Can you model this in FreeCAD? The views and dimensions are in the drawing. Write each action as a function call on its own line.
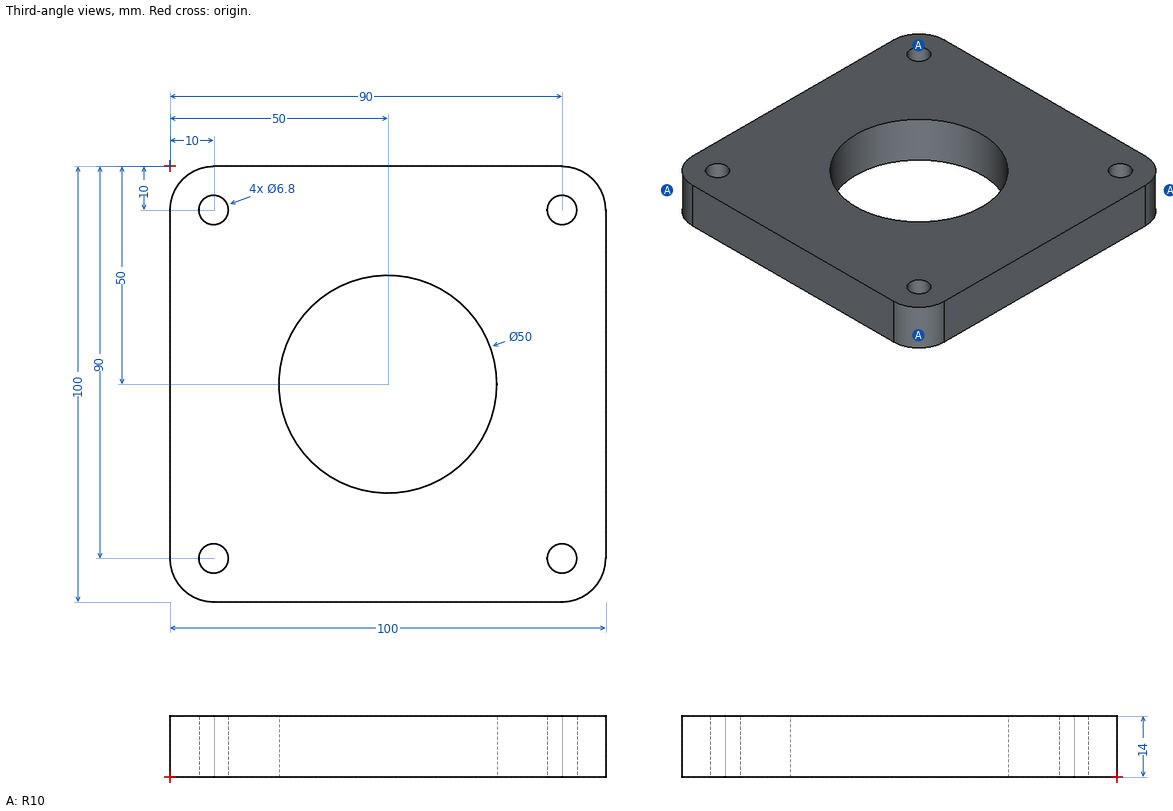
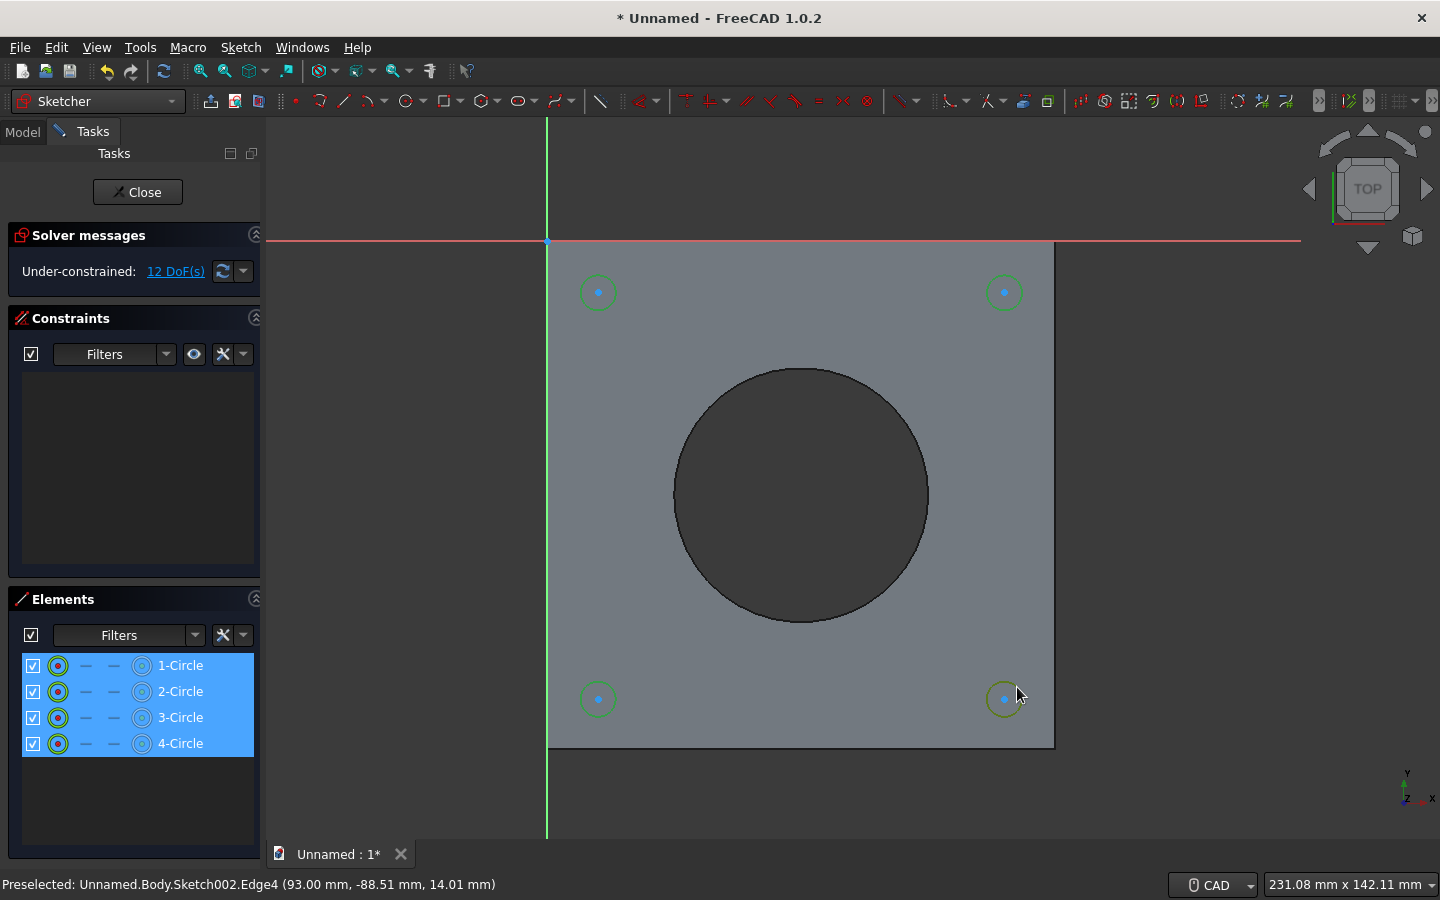
key(e)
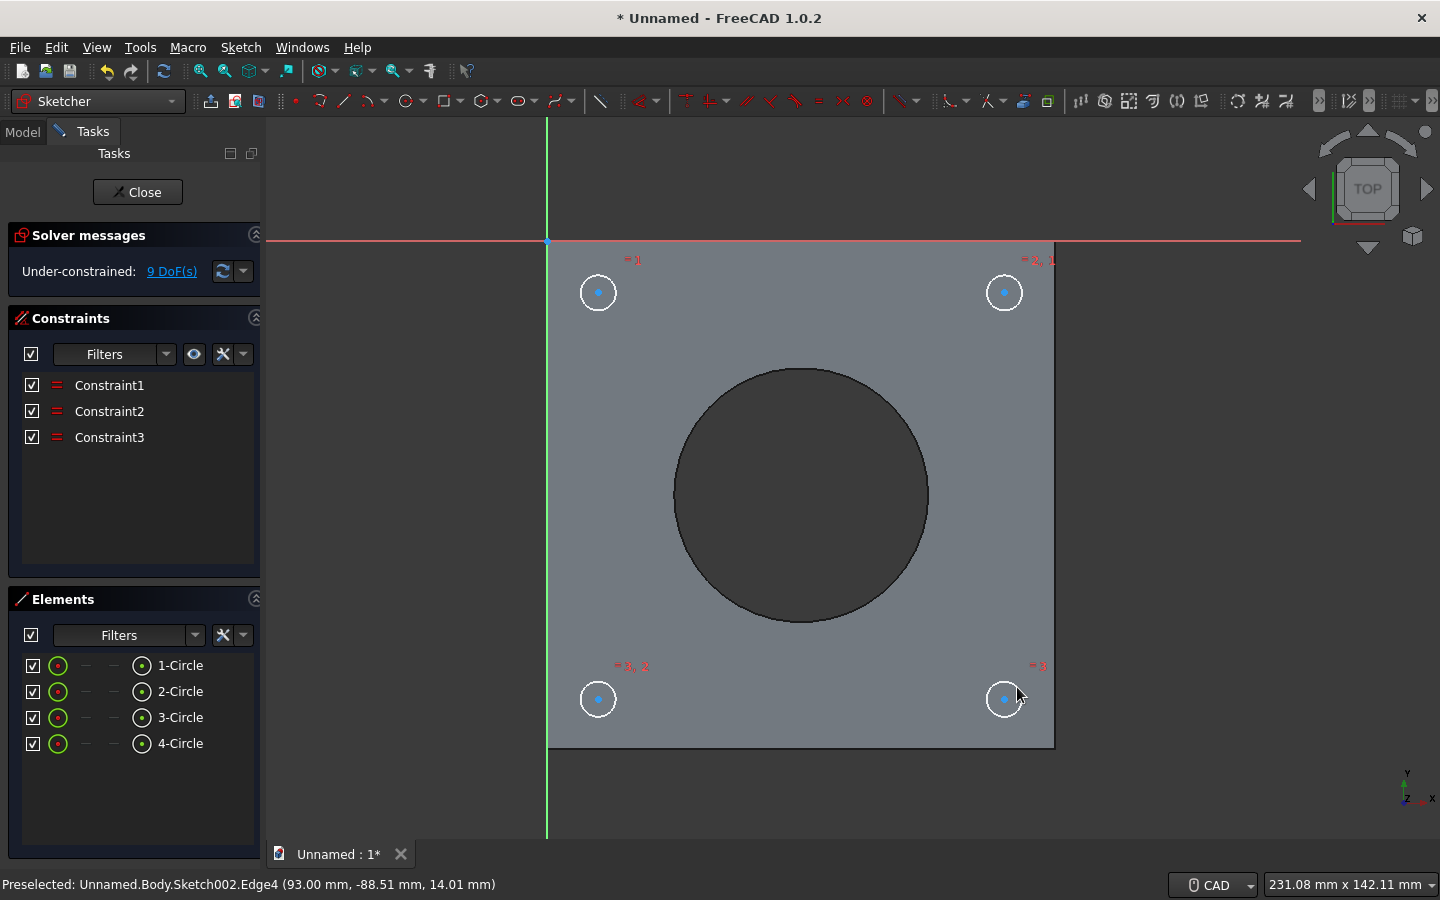
click(598, 293)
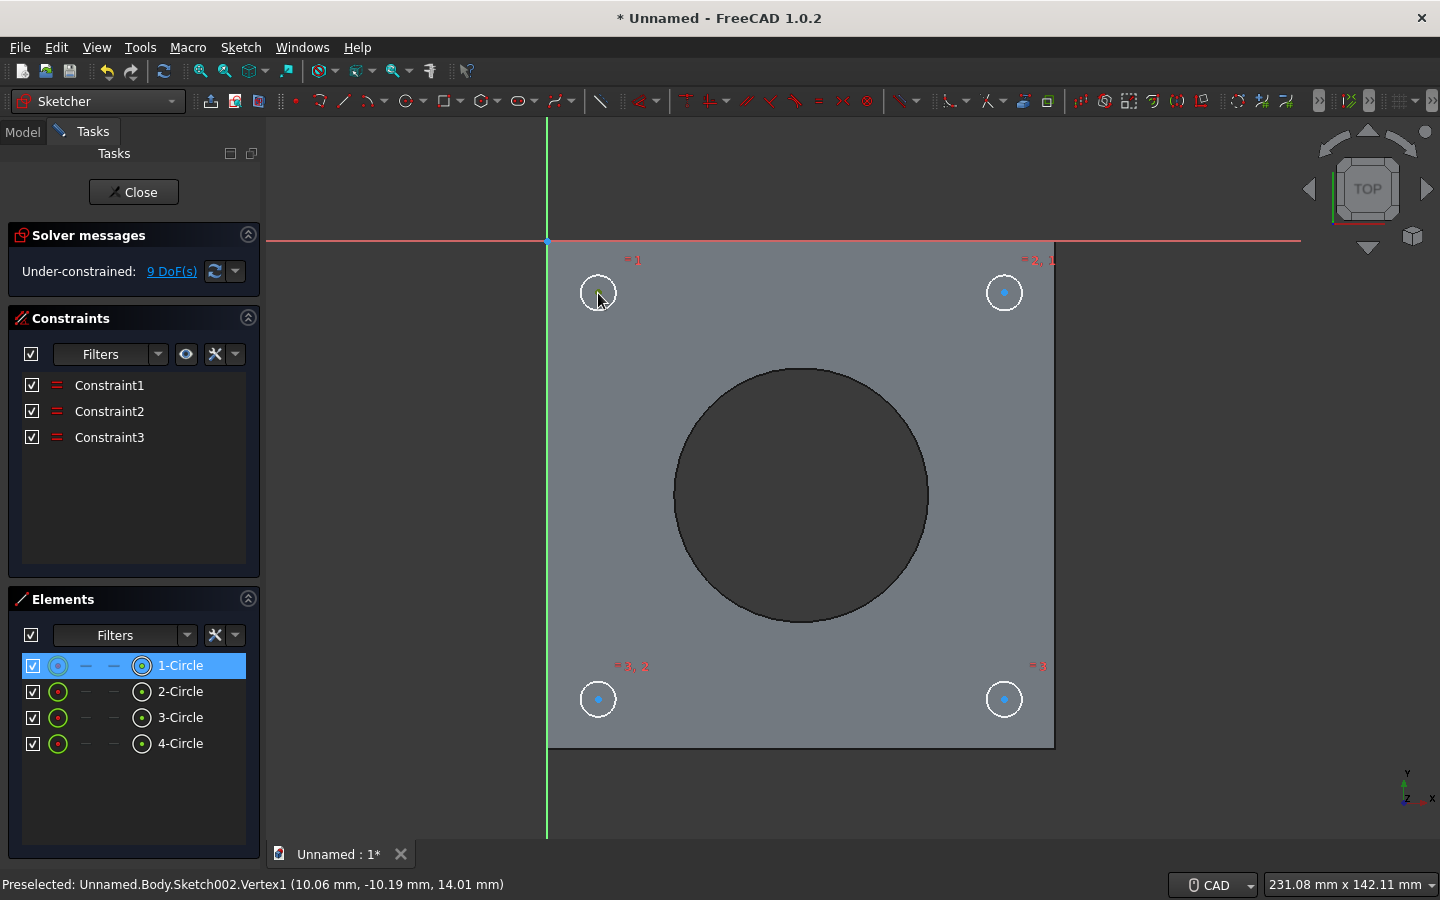
click(1005, 293)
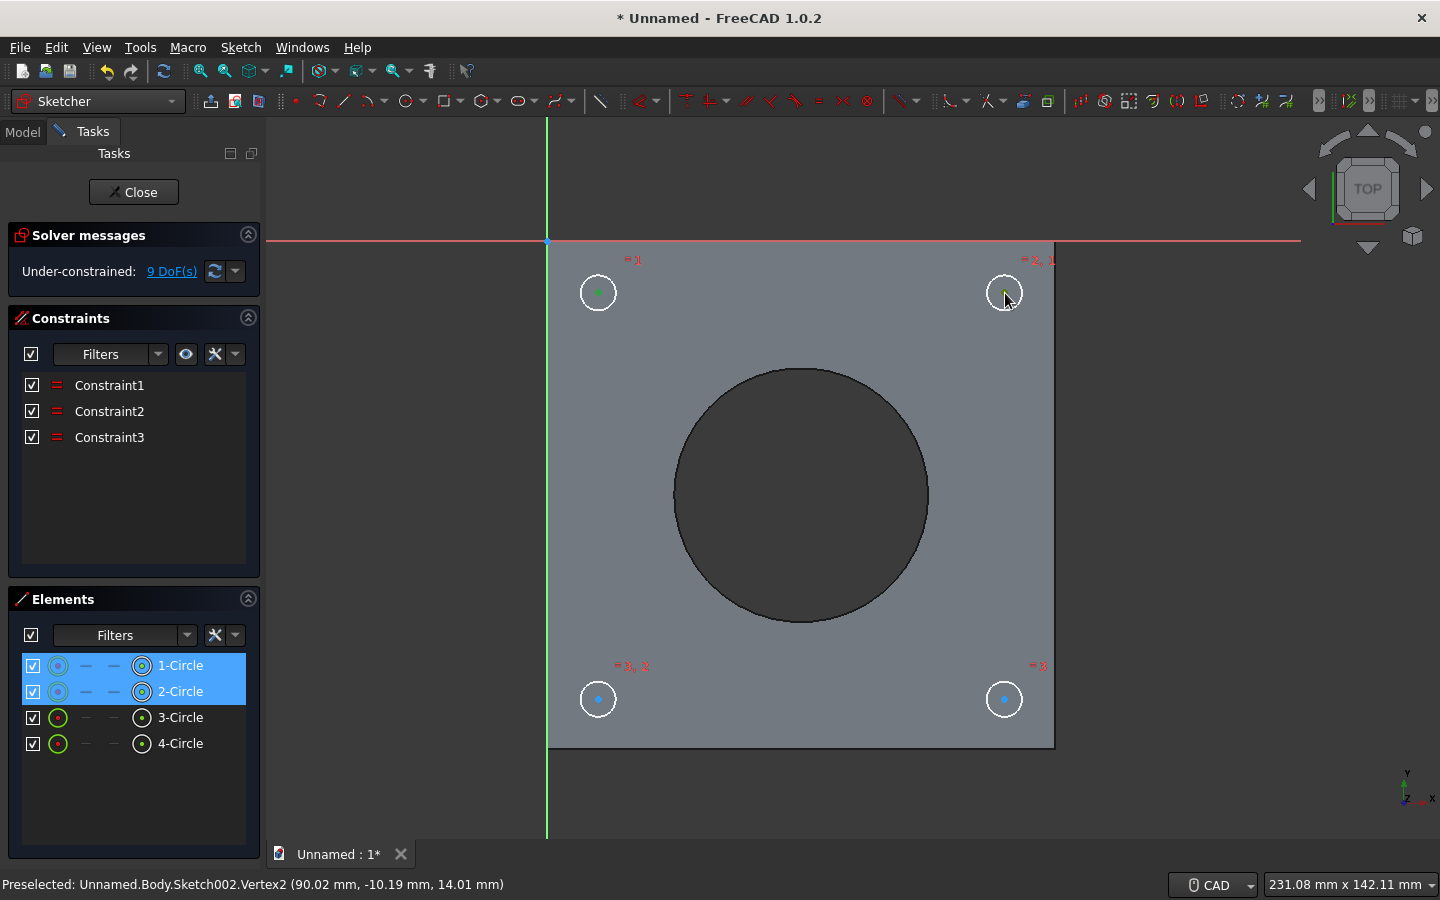
key(h)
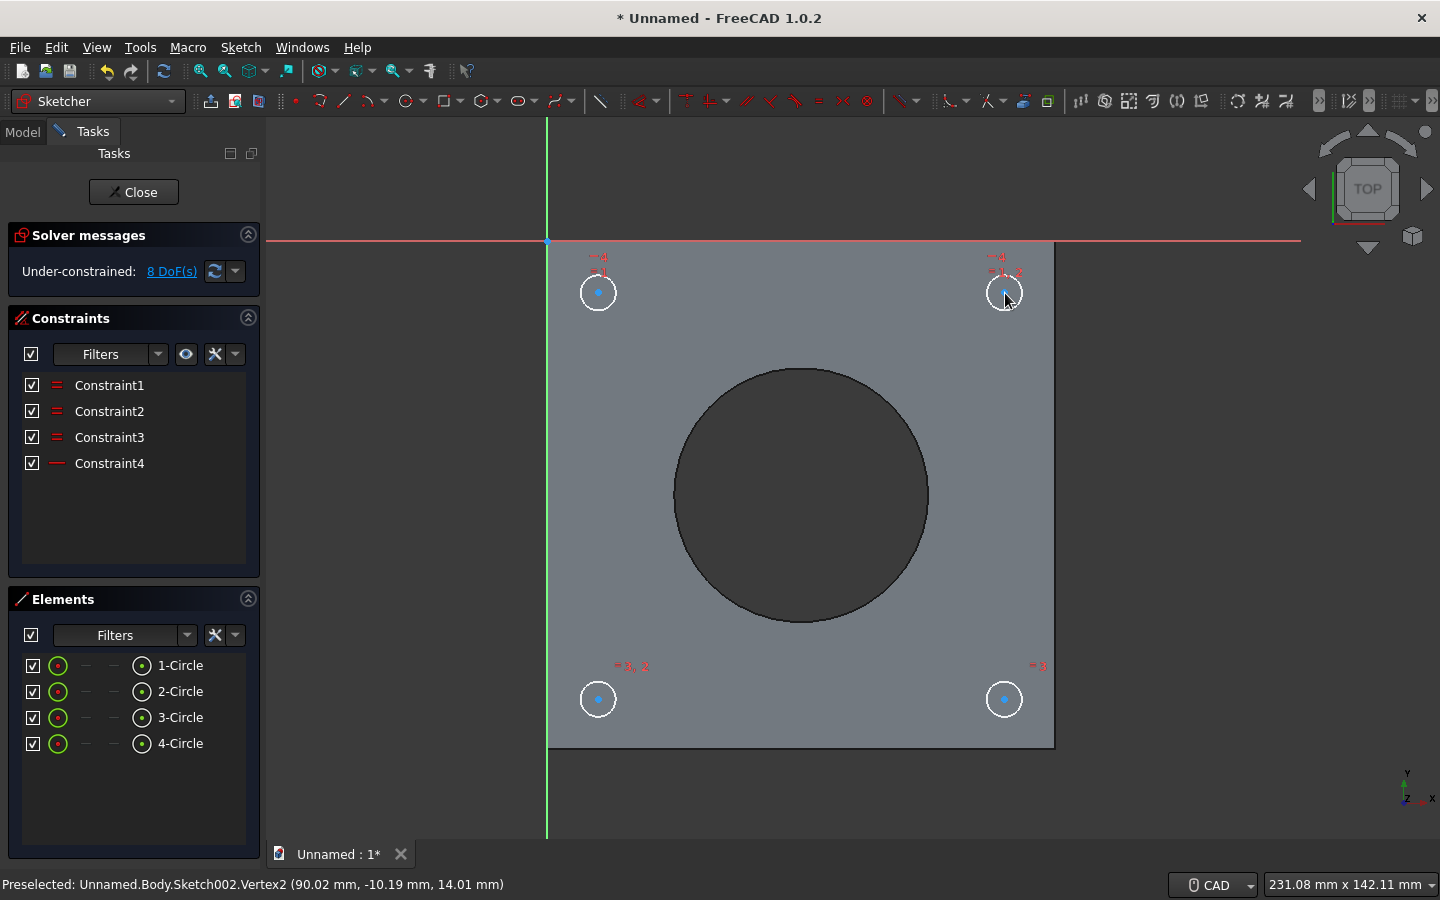
click(598, 293)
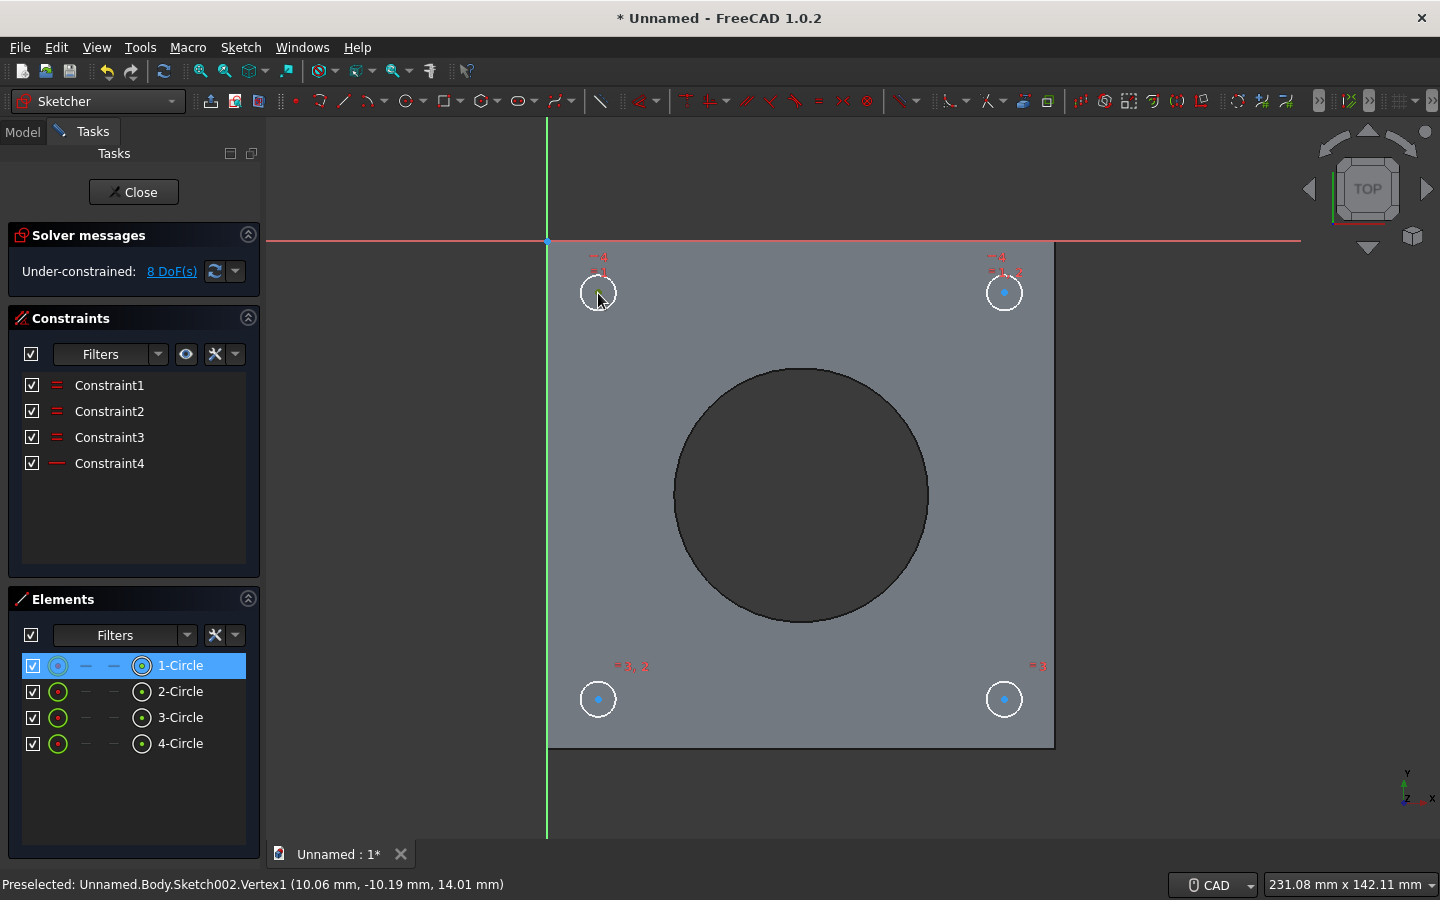
click(598, 699)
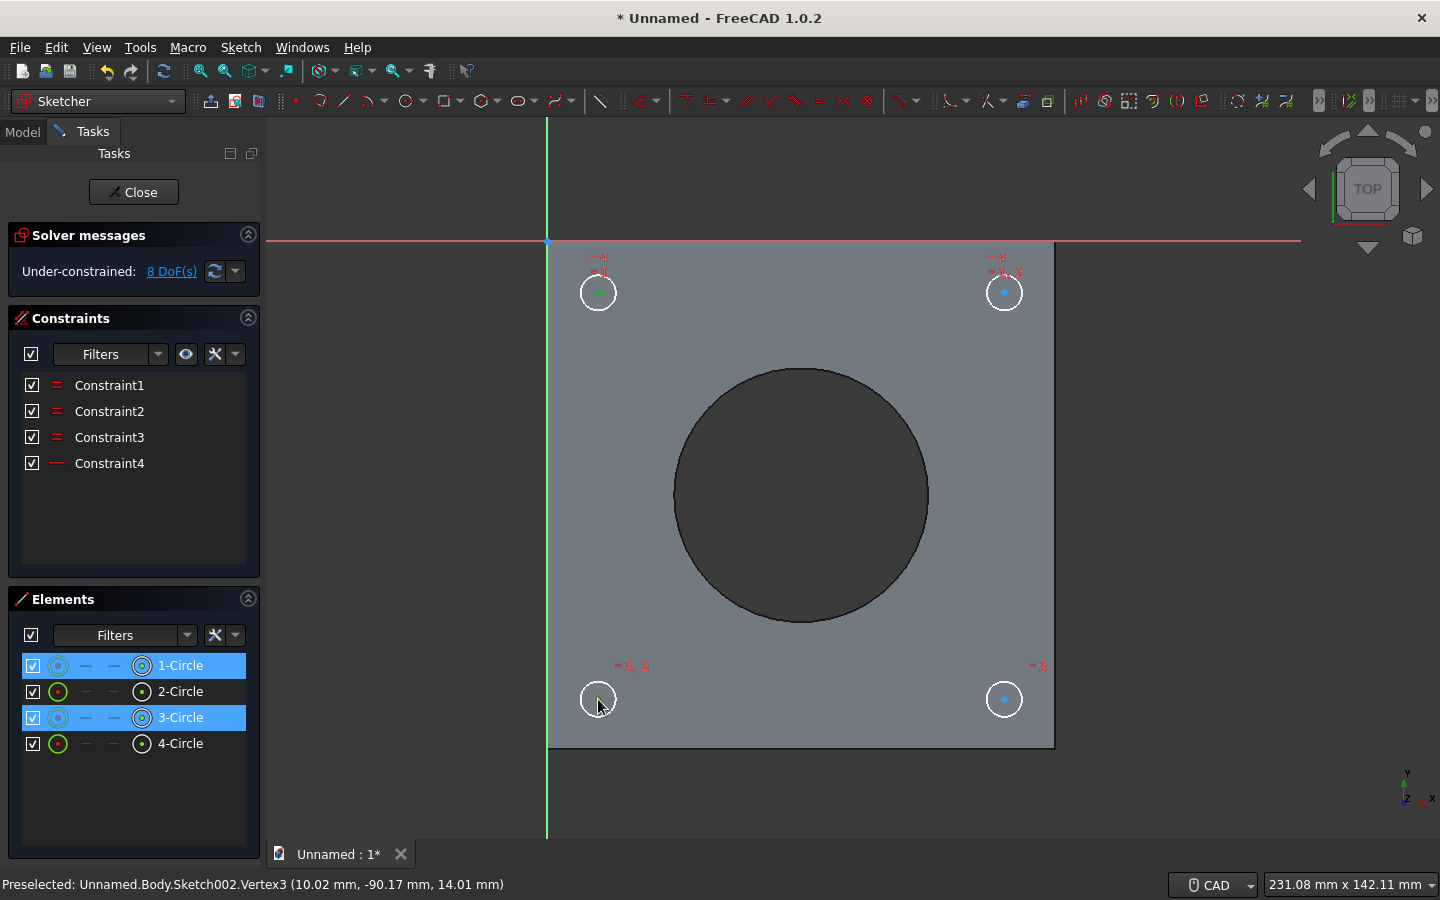
click(728, 102)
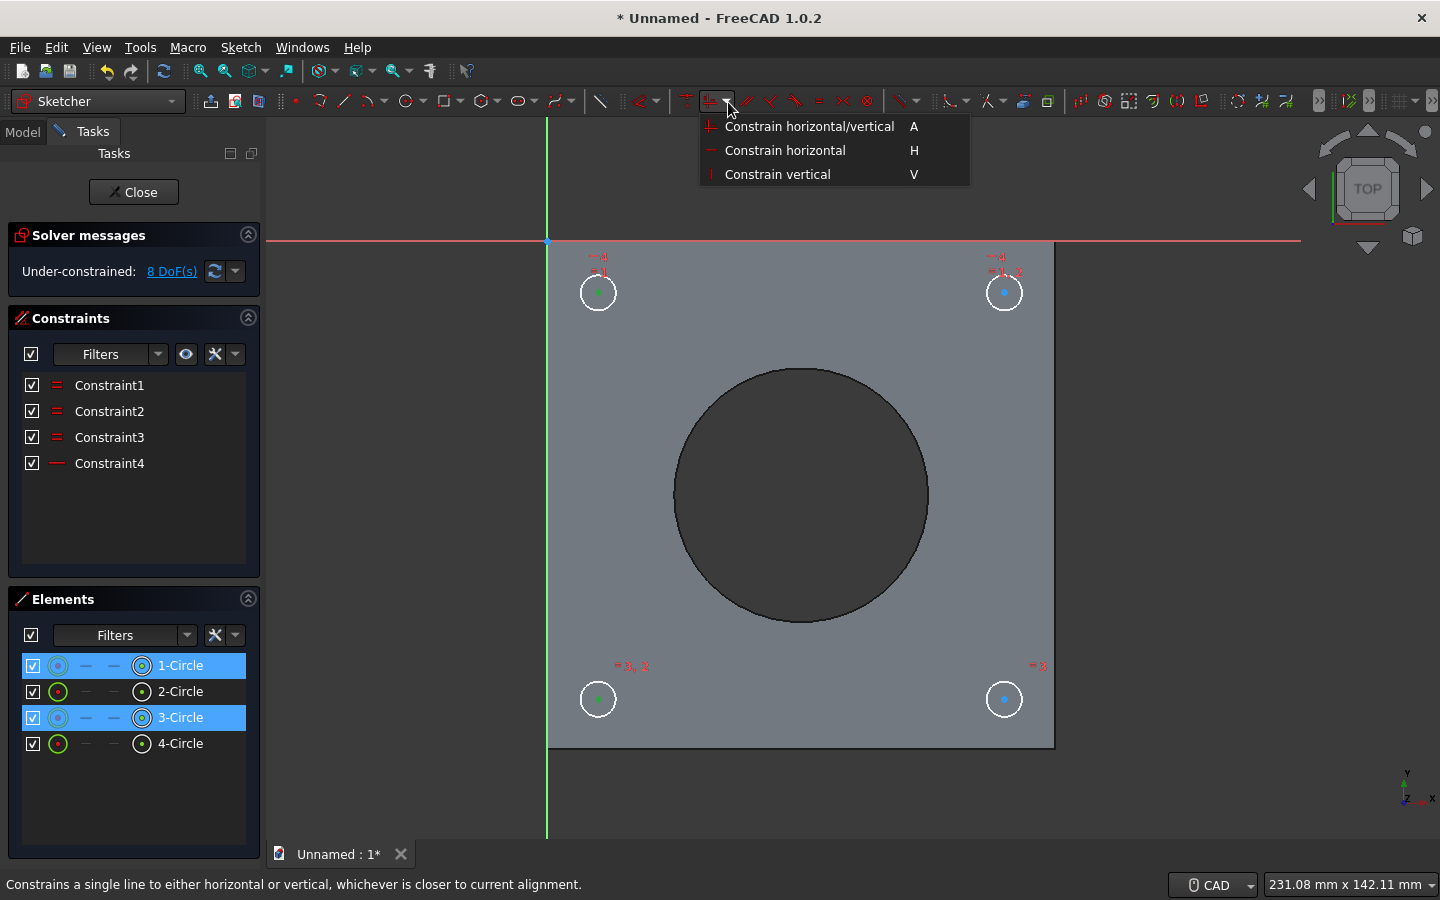
click(835, 174)